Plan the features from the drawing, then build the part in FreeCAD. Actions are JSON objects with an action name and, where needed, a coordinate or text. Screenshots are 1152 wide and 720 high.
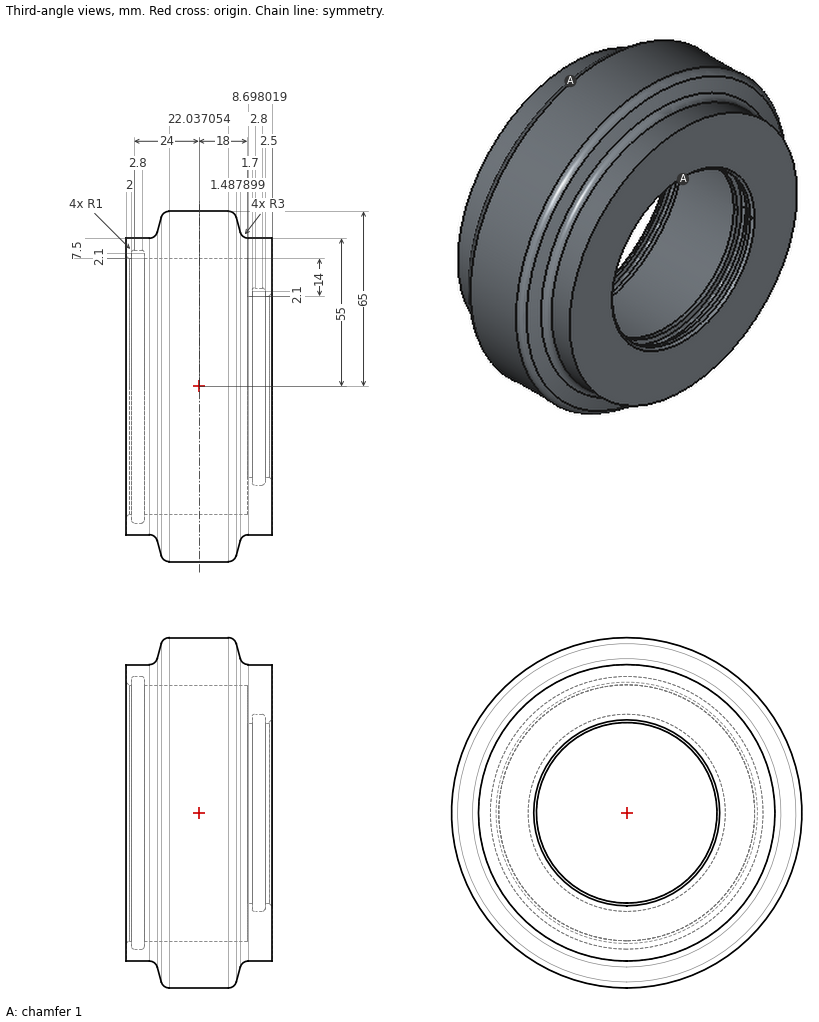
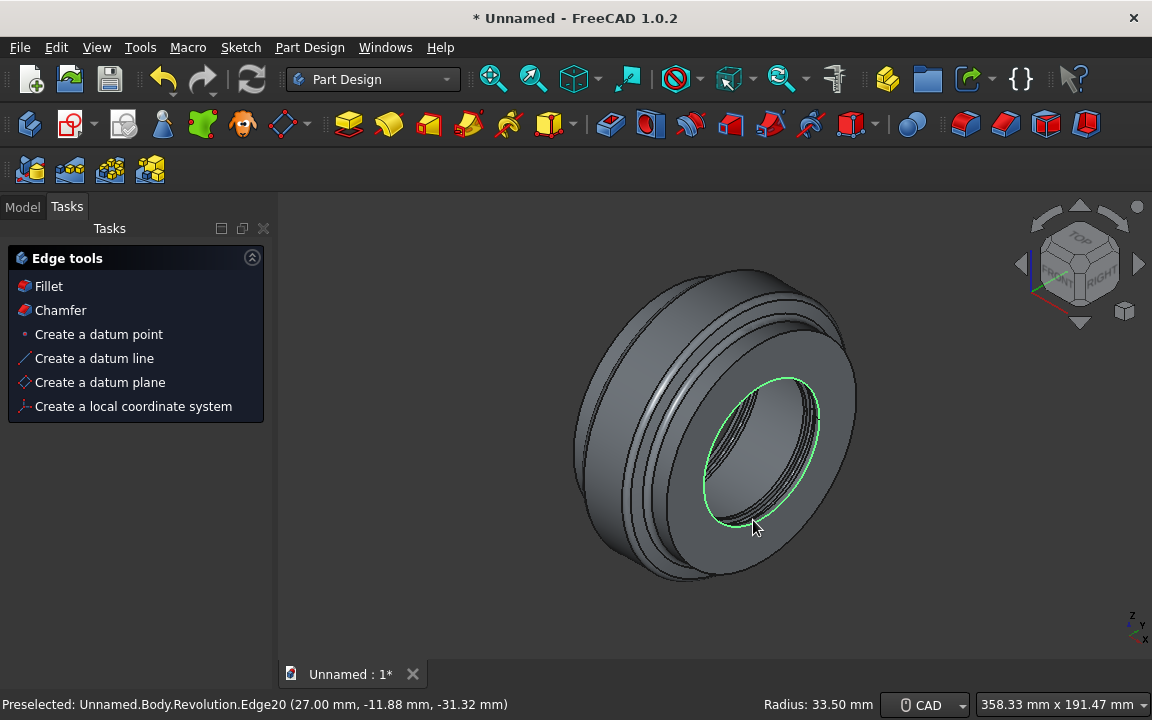
{"action": "key", "text": "2"}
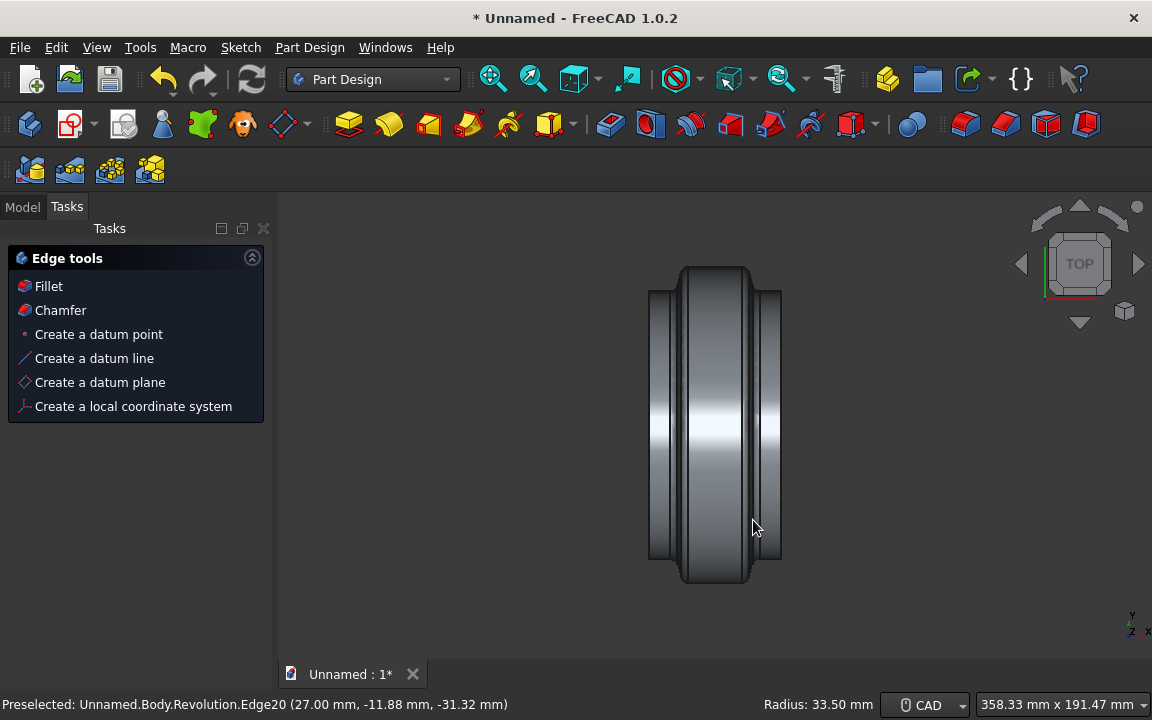
{"action": "key", "text": "1"}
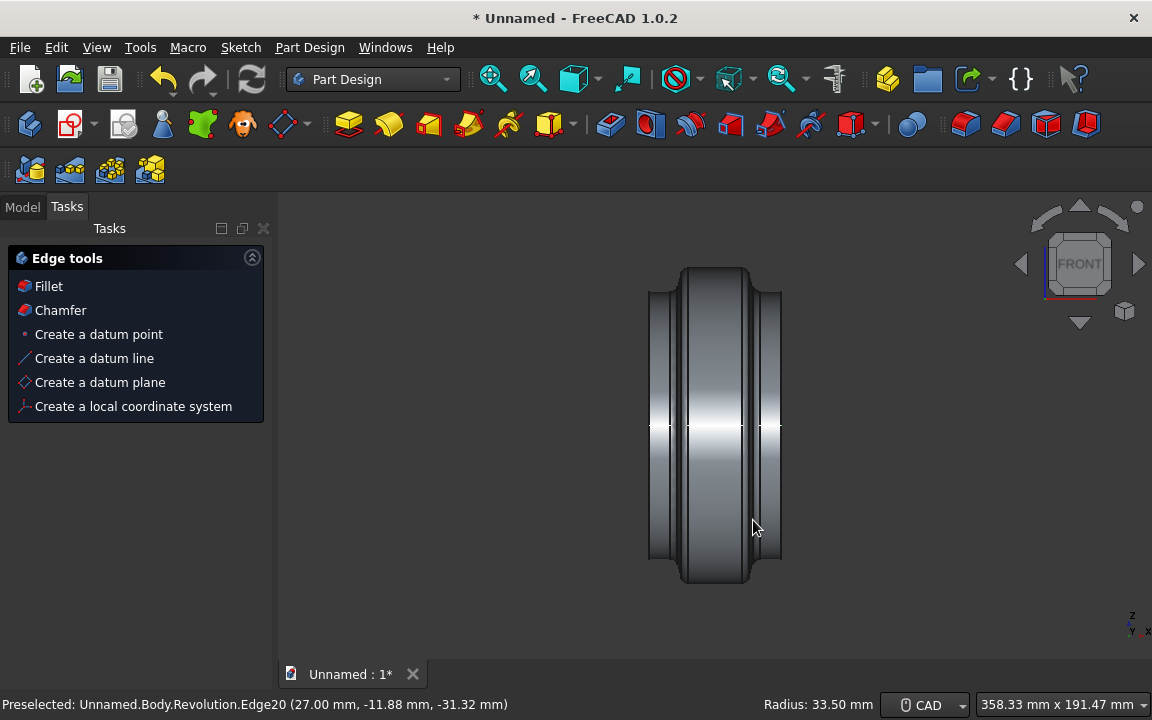
{"action": "key", "text": "3"}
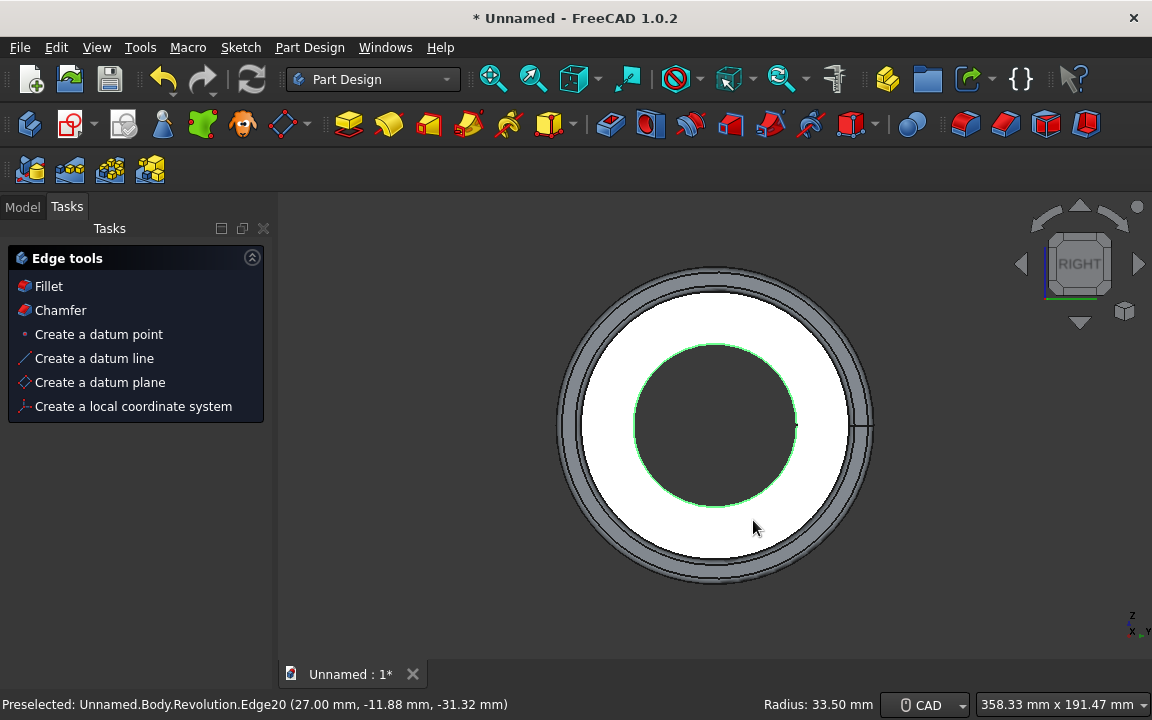
{"action": "key", "text": "5"}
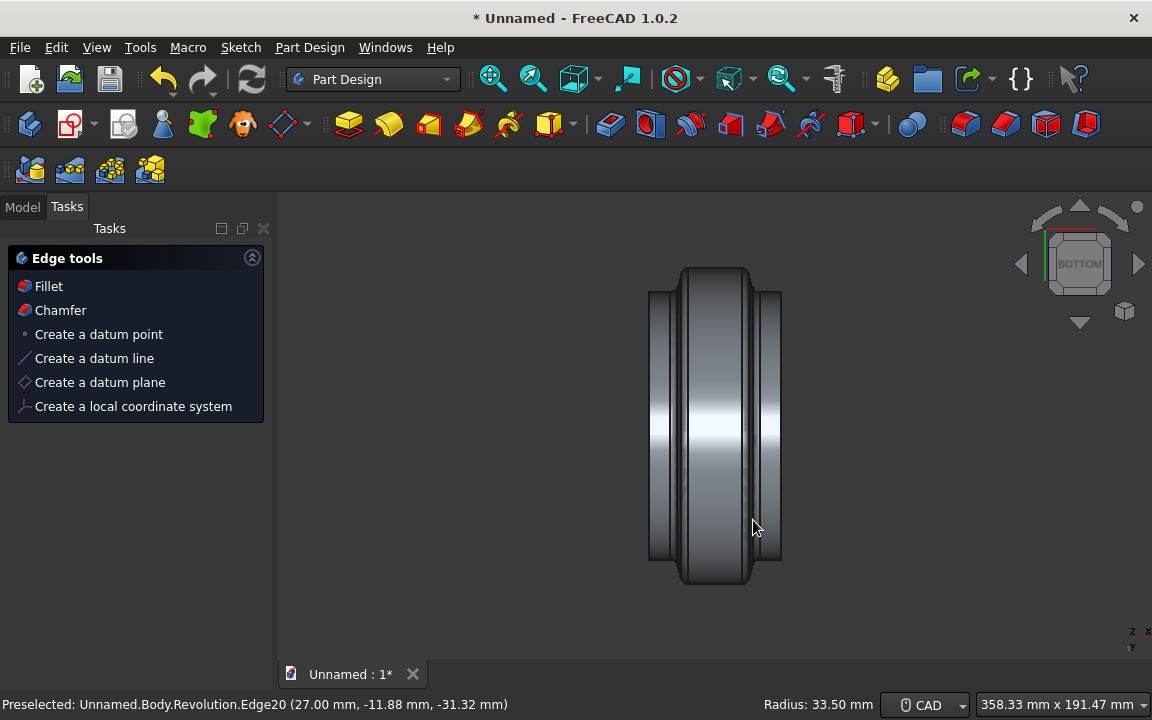
{"action": "key", "text": "4"}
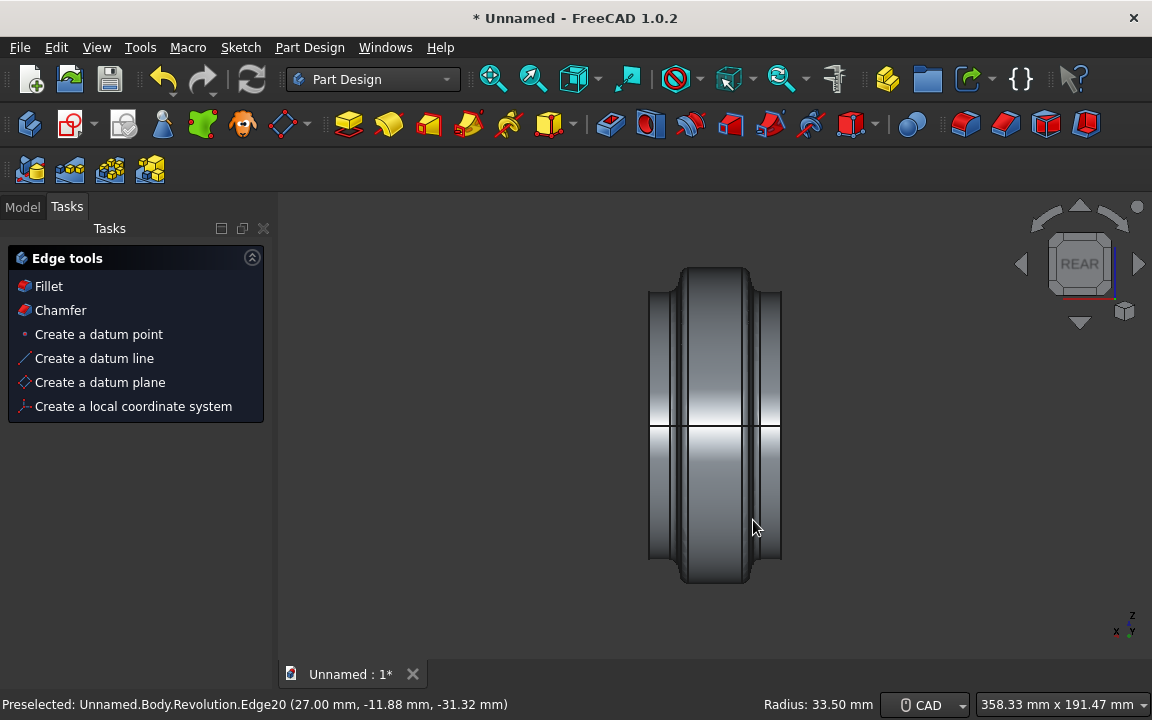
{"action": "key", "text": "6"}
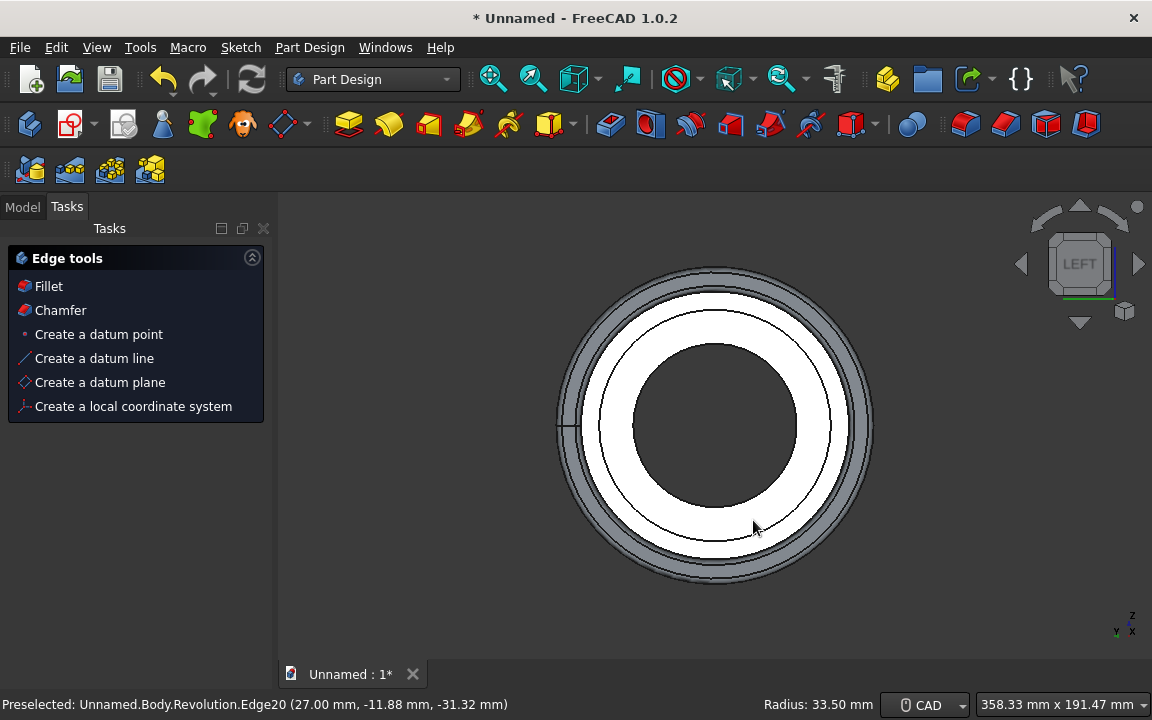
{"action": "left_click", "coordinate": [831, 424], "text": "ctrl"}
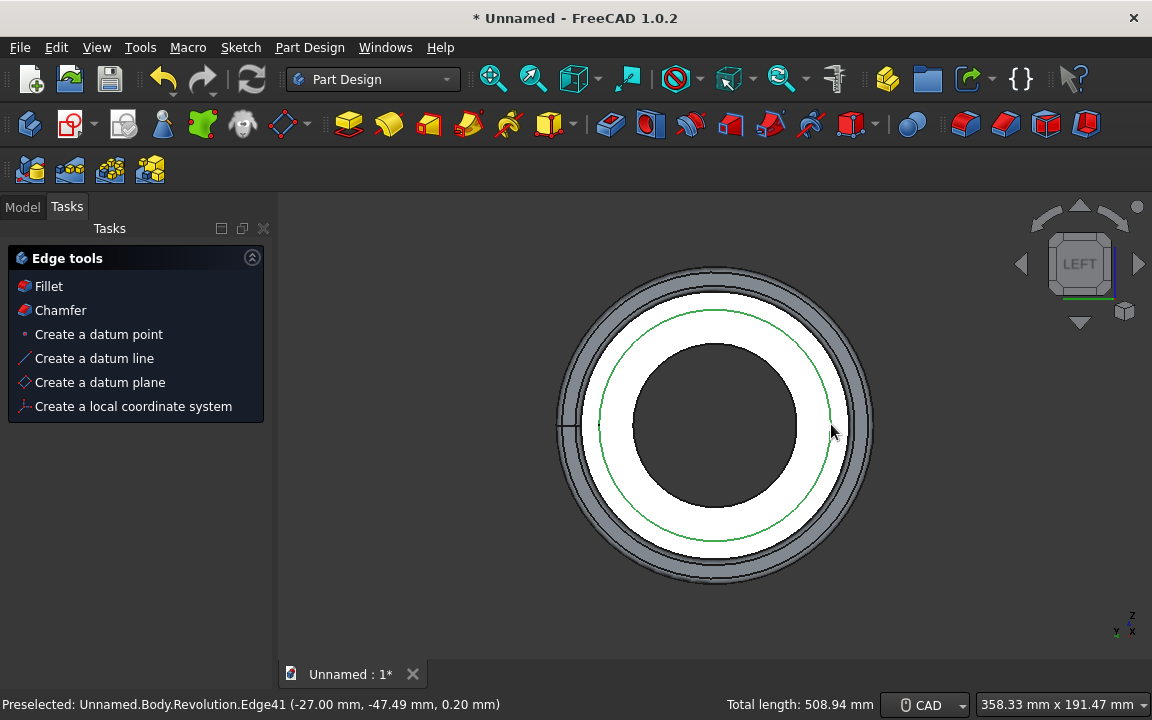
{"action": "left_click", "coordinate": [1006, 124]}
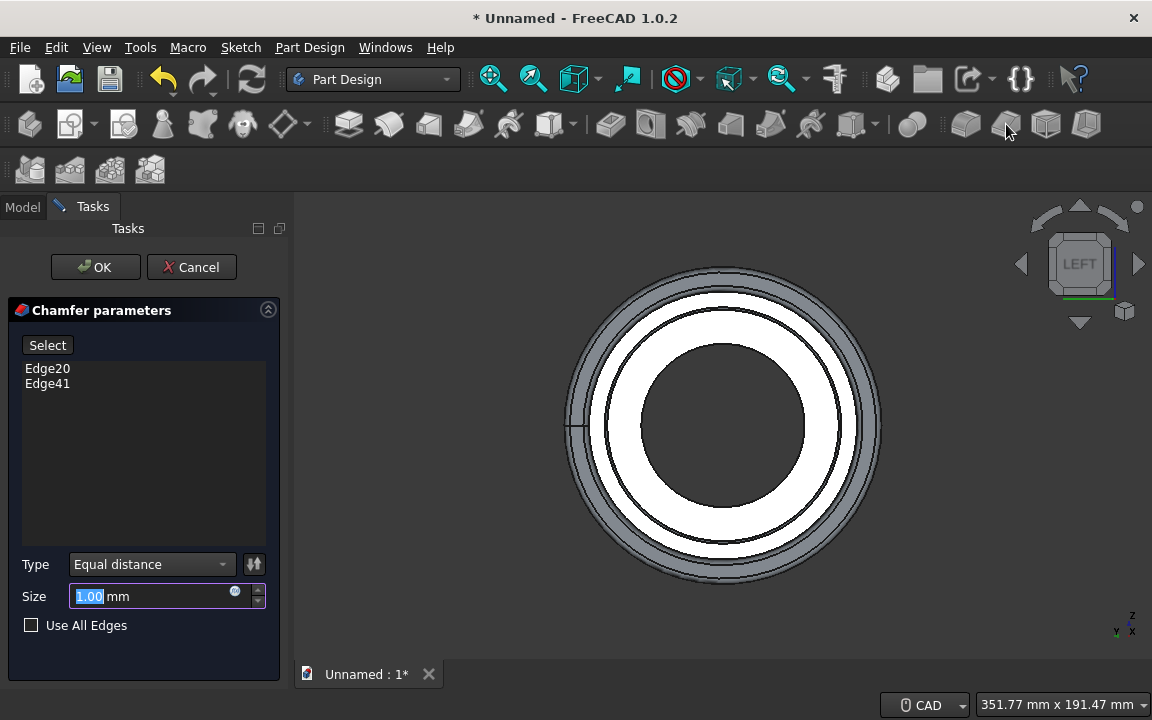
{"action": "type", "text": "1"}
{"action": "key", "text": "Tab"}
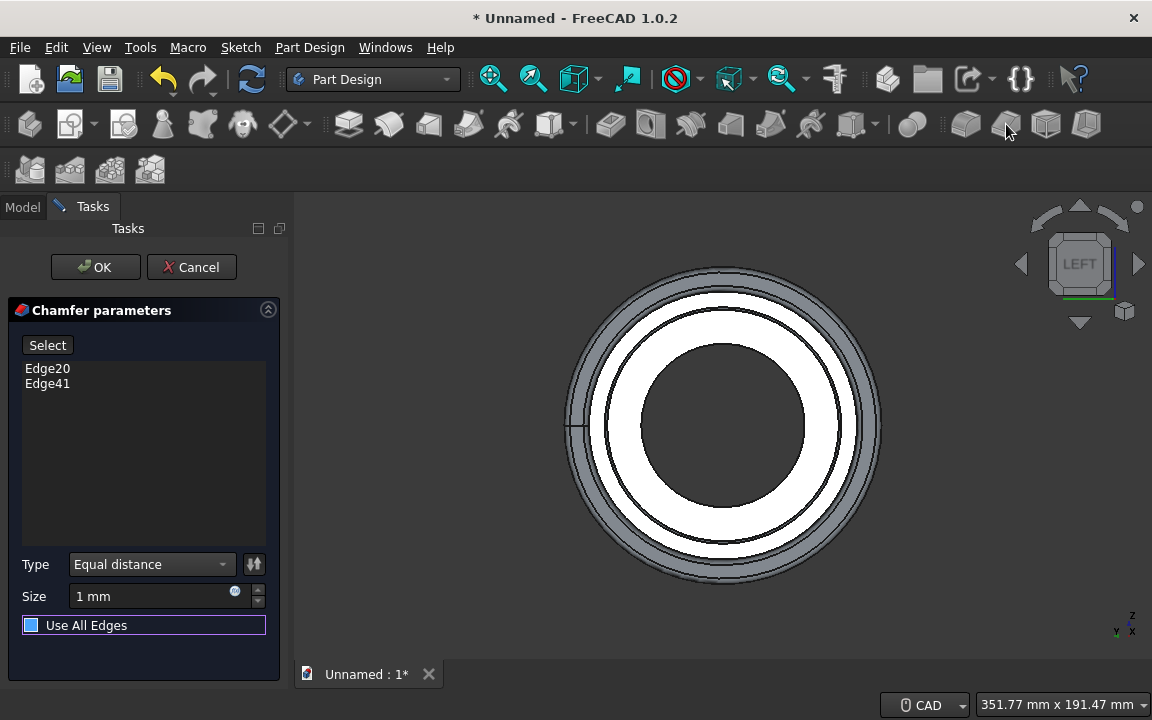
{"action": "left_click", "coordinate": [96, 267]}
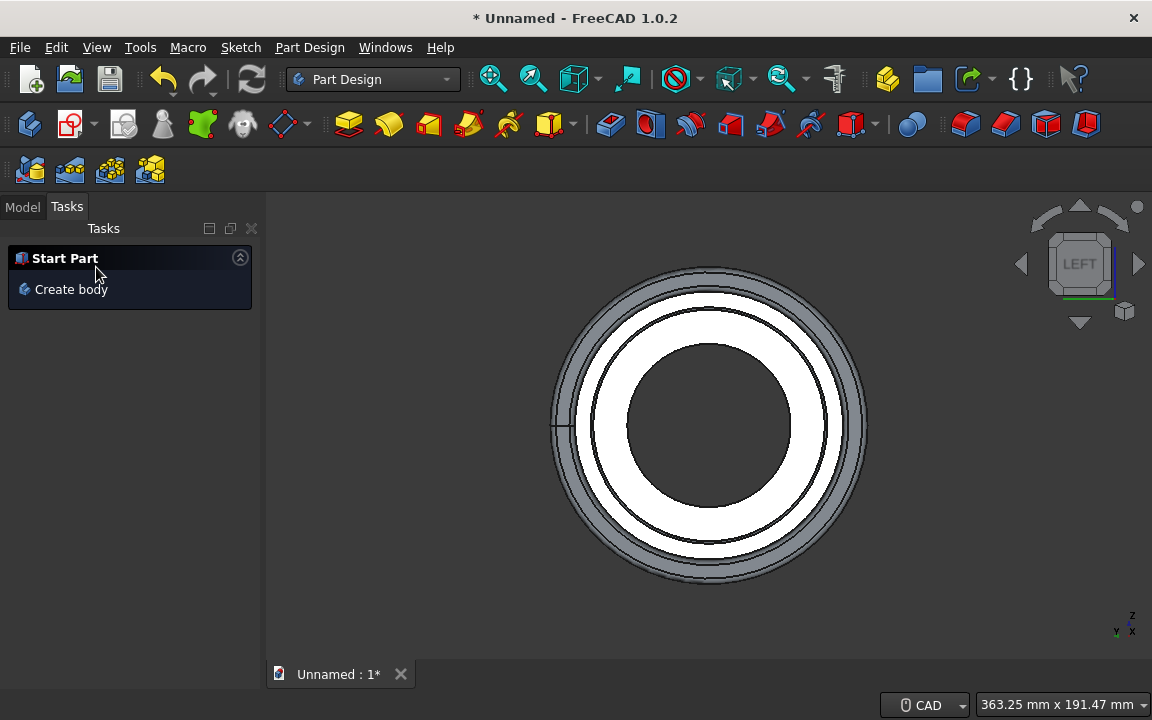
{"action": "key", "text": "0"}